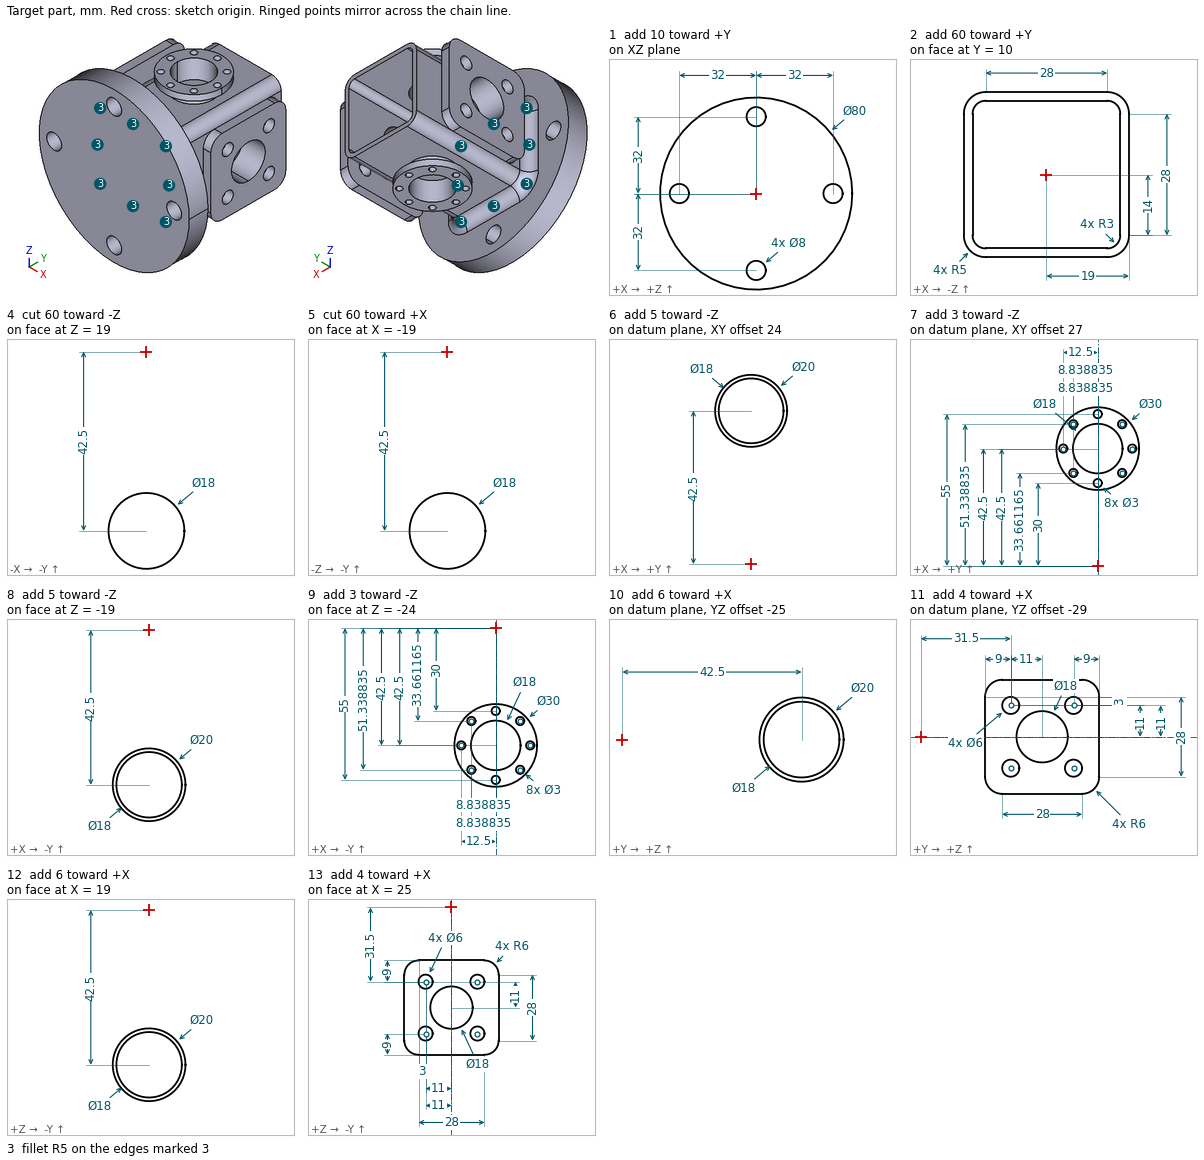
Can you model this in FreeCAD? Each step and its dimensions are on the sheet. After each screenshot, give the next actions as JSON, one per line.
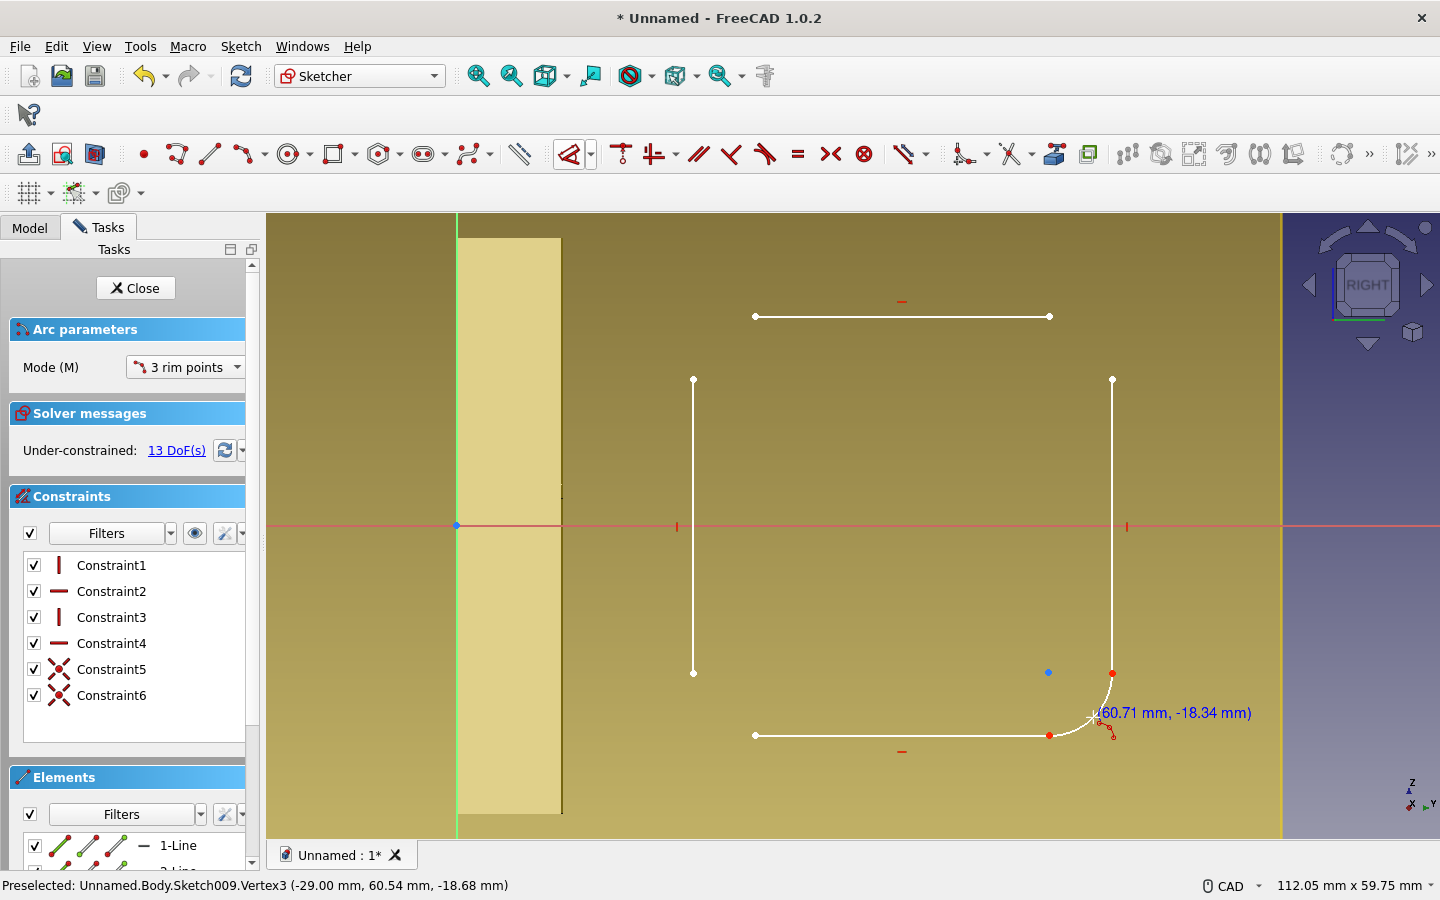
{"action": "left_click", "coordinate": [755, 736]}
{"action": "left_click", "coordinate": [693, 674]}
{"action": "left_click", "coordinate": [711, 717]}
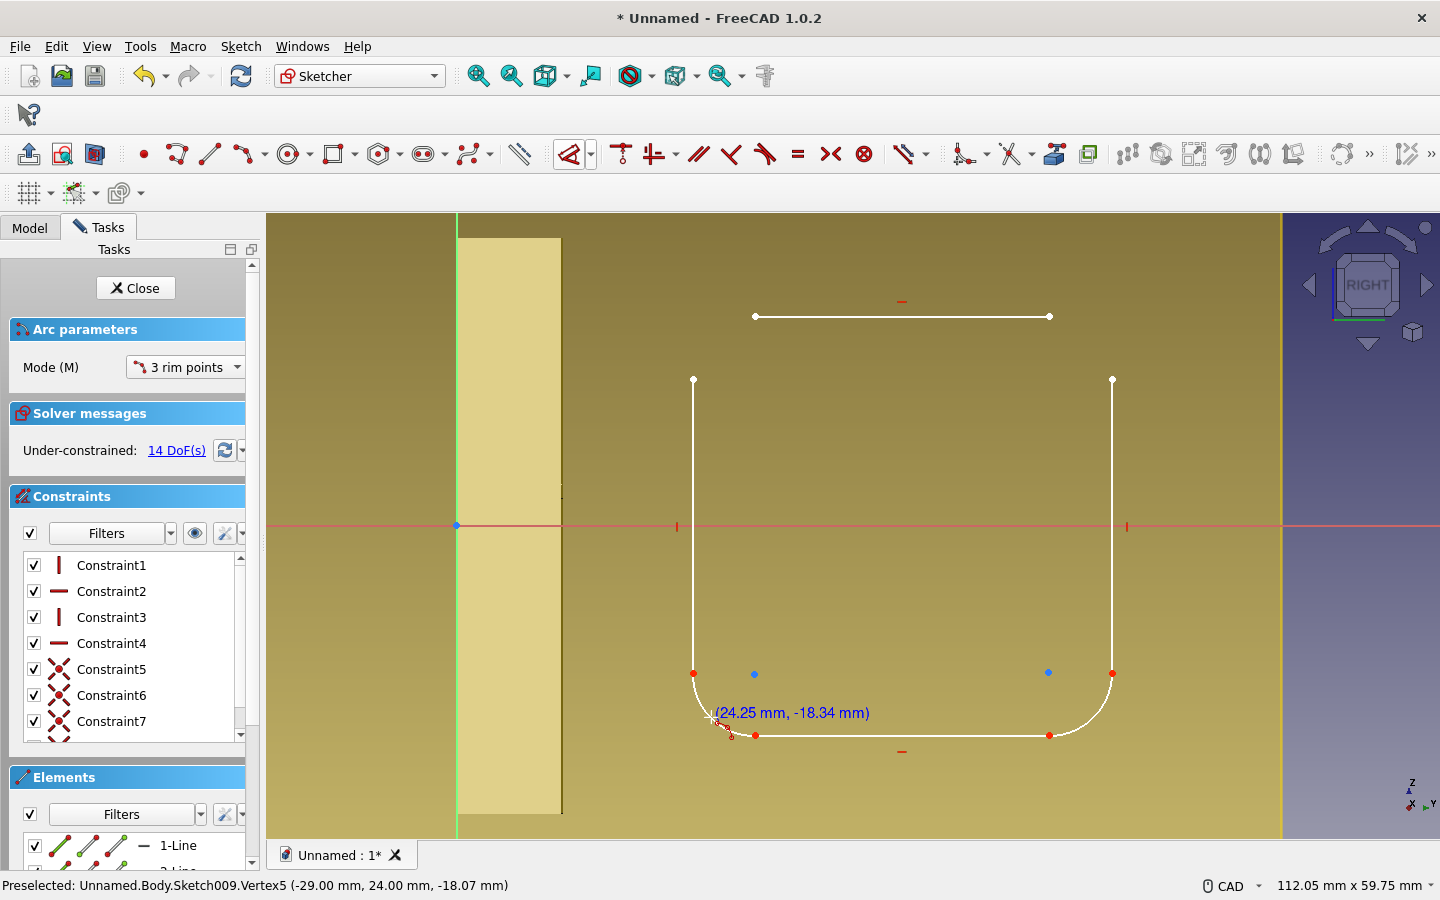
{"action": "left_click", "coordinate": [693, 380]}
{"action": "left_click", "coordinate": [755, 317]}
{"action": "left_click", "coordinate": [711, 335]}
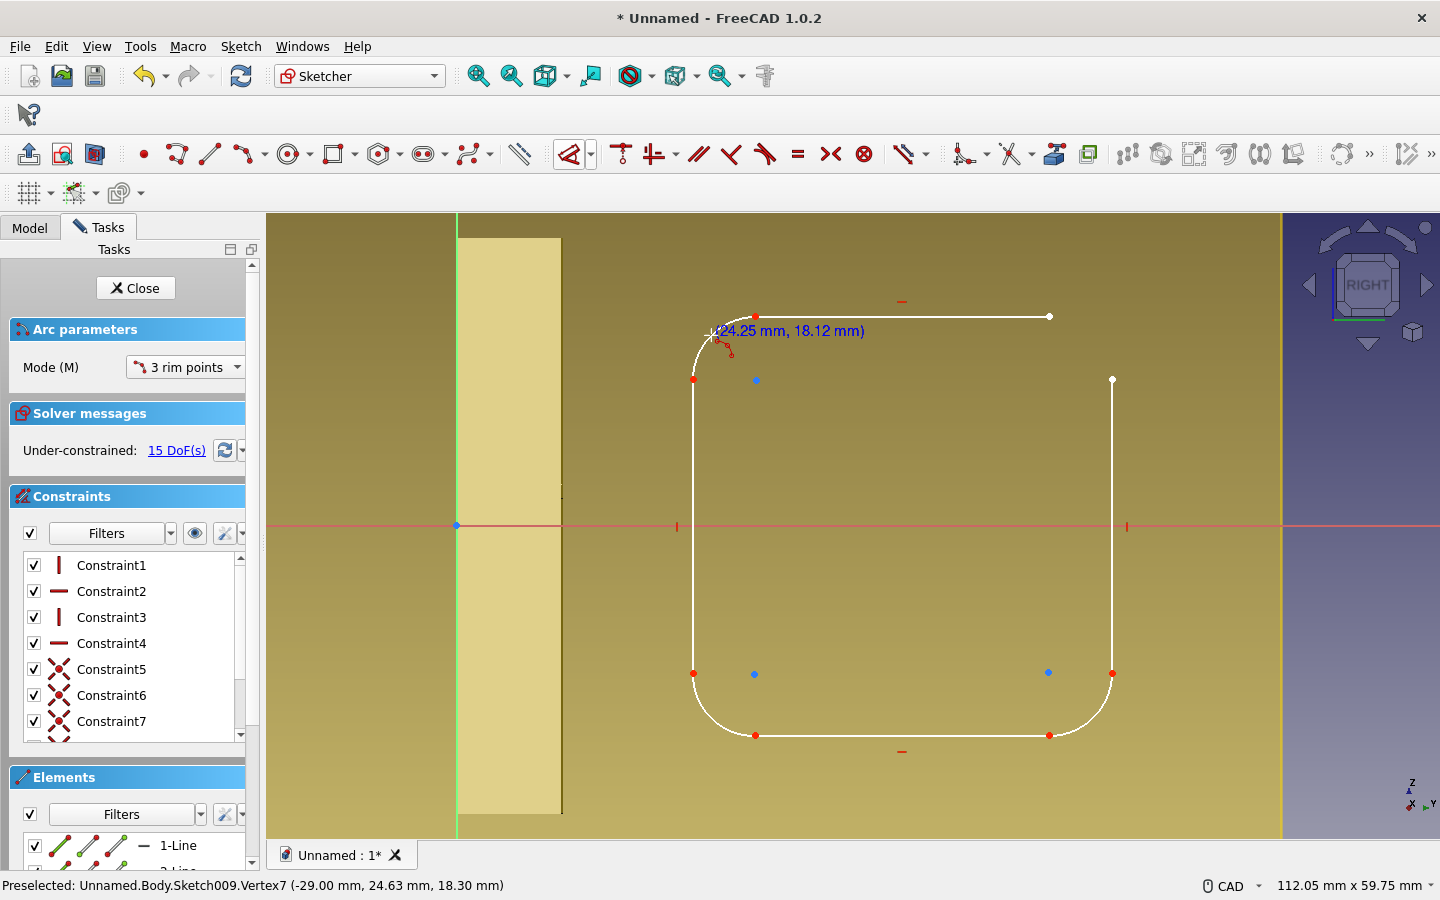
{"action": "left_click", "coordinate": [1049, 317]}
{"action": "left_click", "coordinate": [1112, 380]}
{"action": "left_click", "coordinate": [1093, 335]}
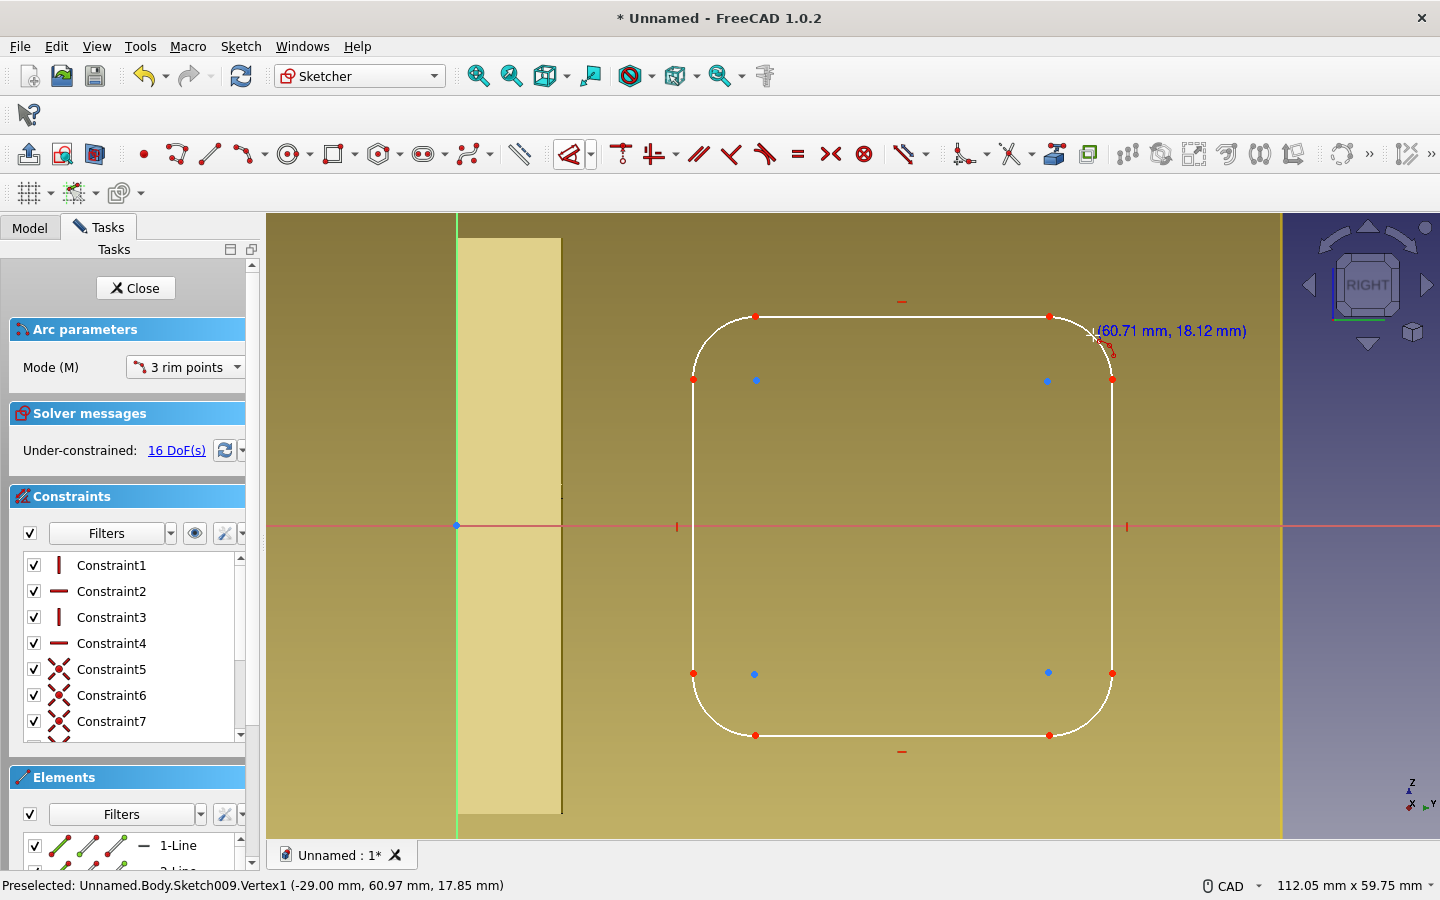
{"action": "key", "text": "g c"}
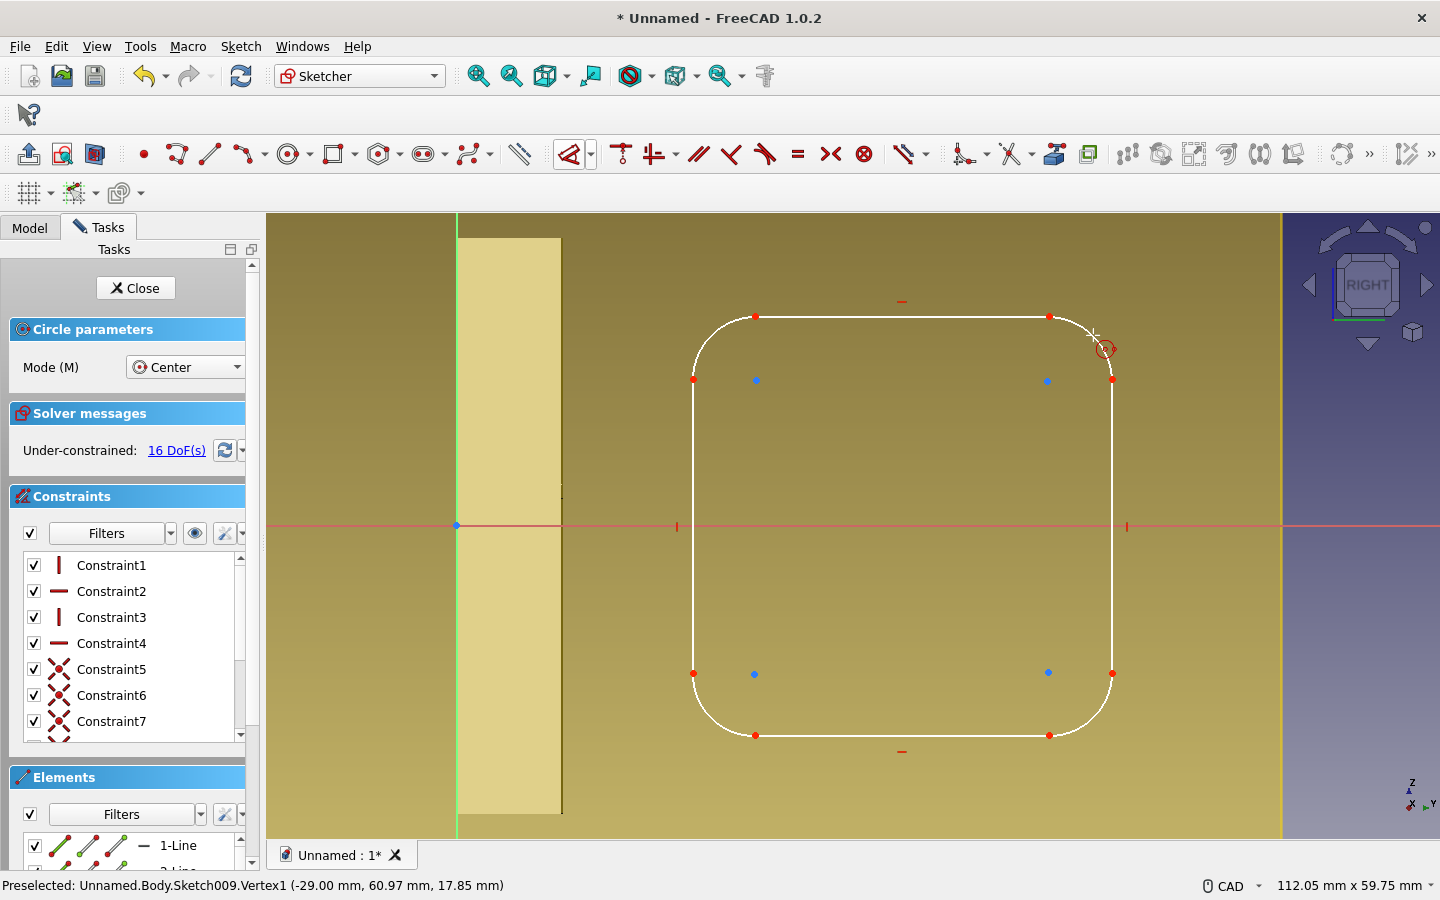
{"action": "left_click", "coordinate": [787, 411]}
{"action": "mouse_move", "coordinate": [809, 388]}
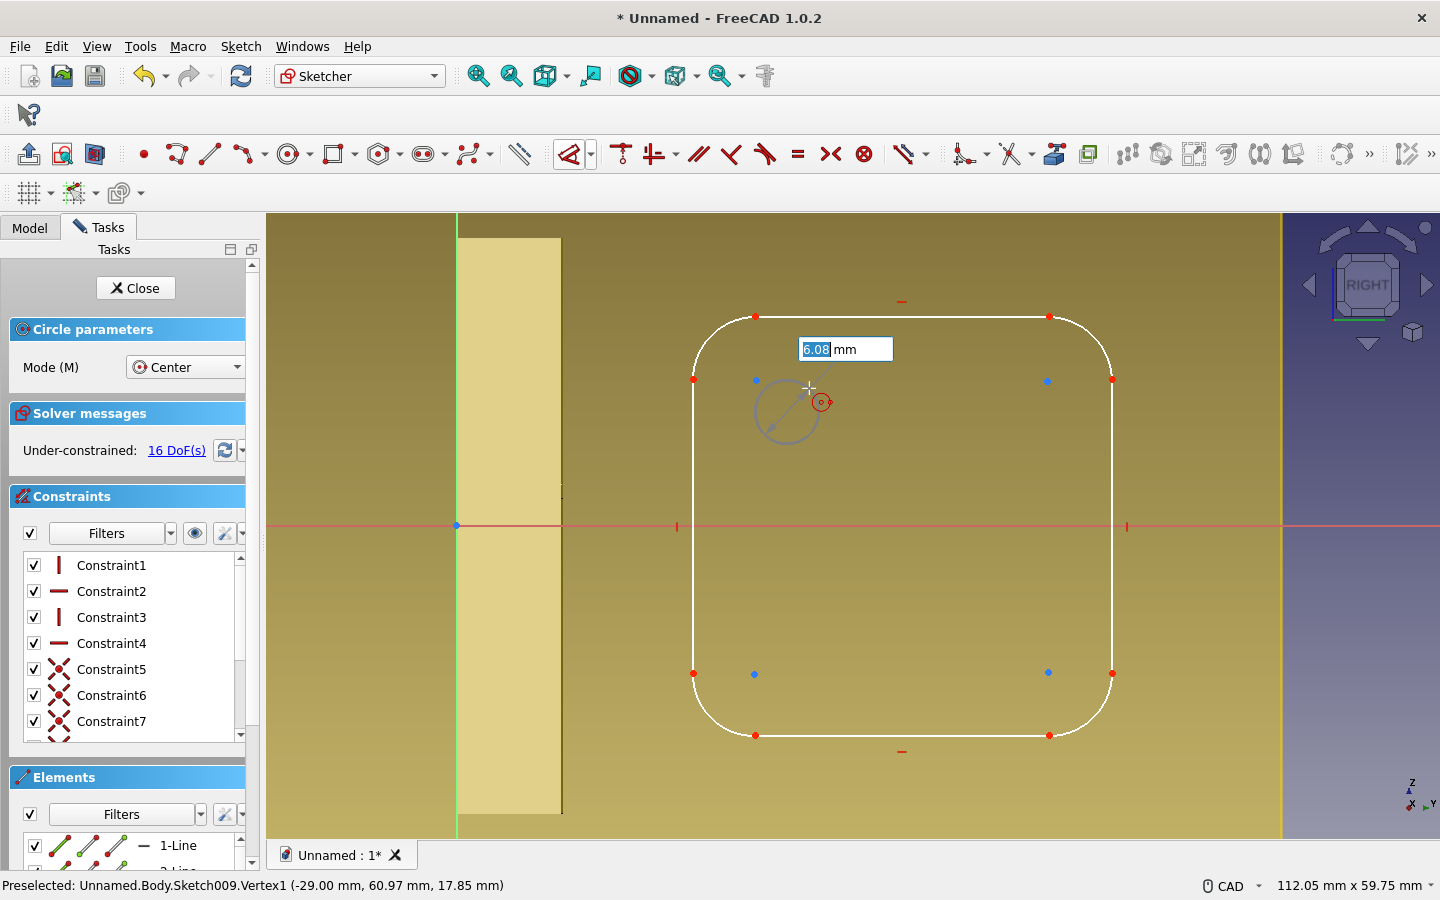
{"action": "type", "text": "6"}
{"action": "key", "text": "Return"}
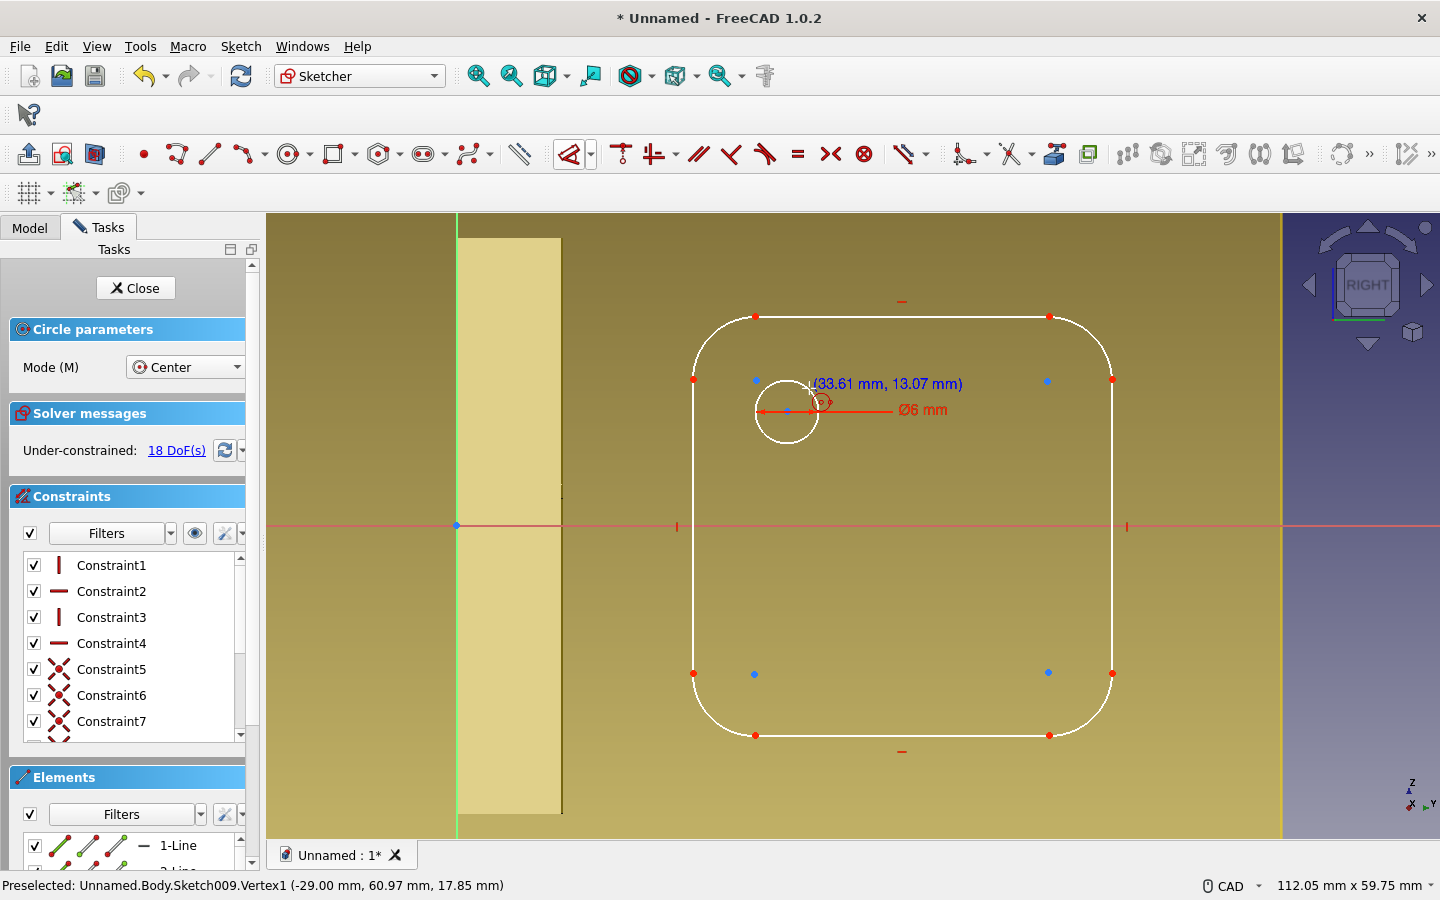
{"action": "left_click", "coordinate": [787, 641]}
{"action": "mouse_move", "coordinate": [809, 619]}